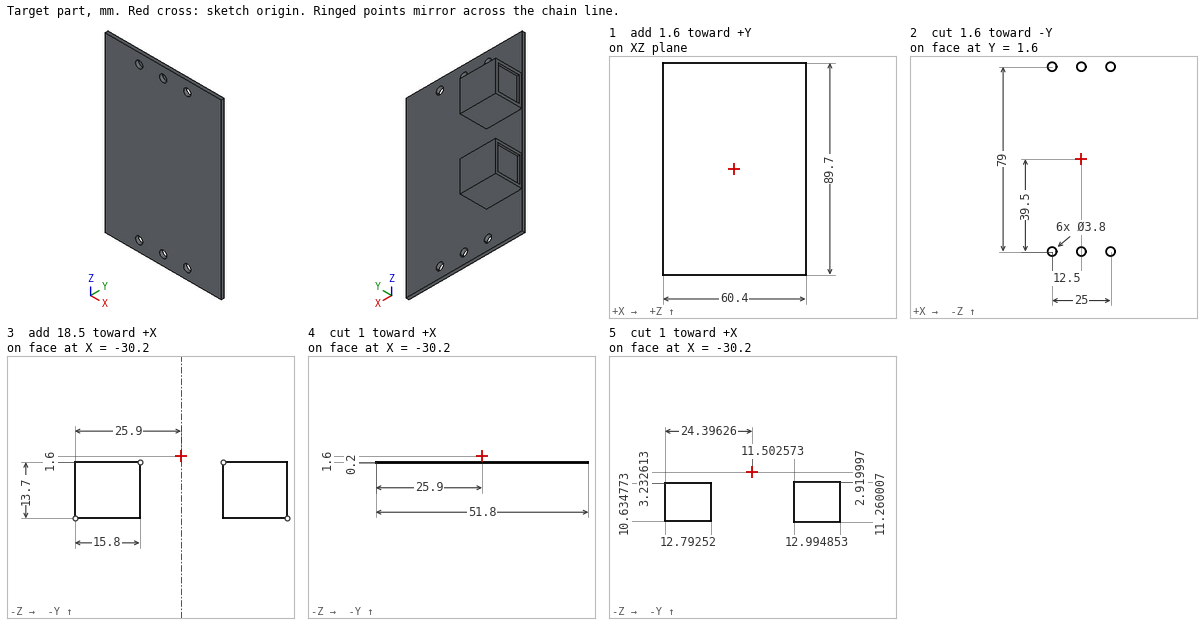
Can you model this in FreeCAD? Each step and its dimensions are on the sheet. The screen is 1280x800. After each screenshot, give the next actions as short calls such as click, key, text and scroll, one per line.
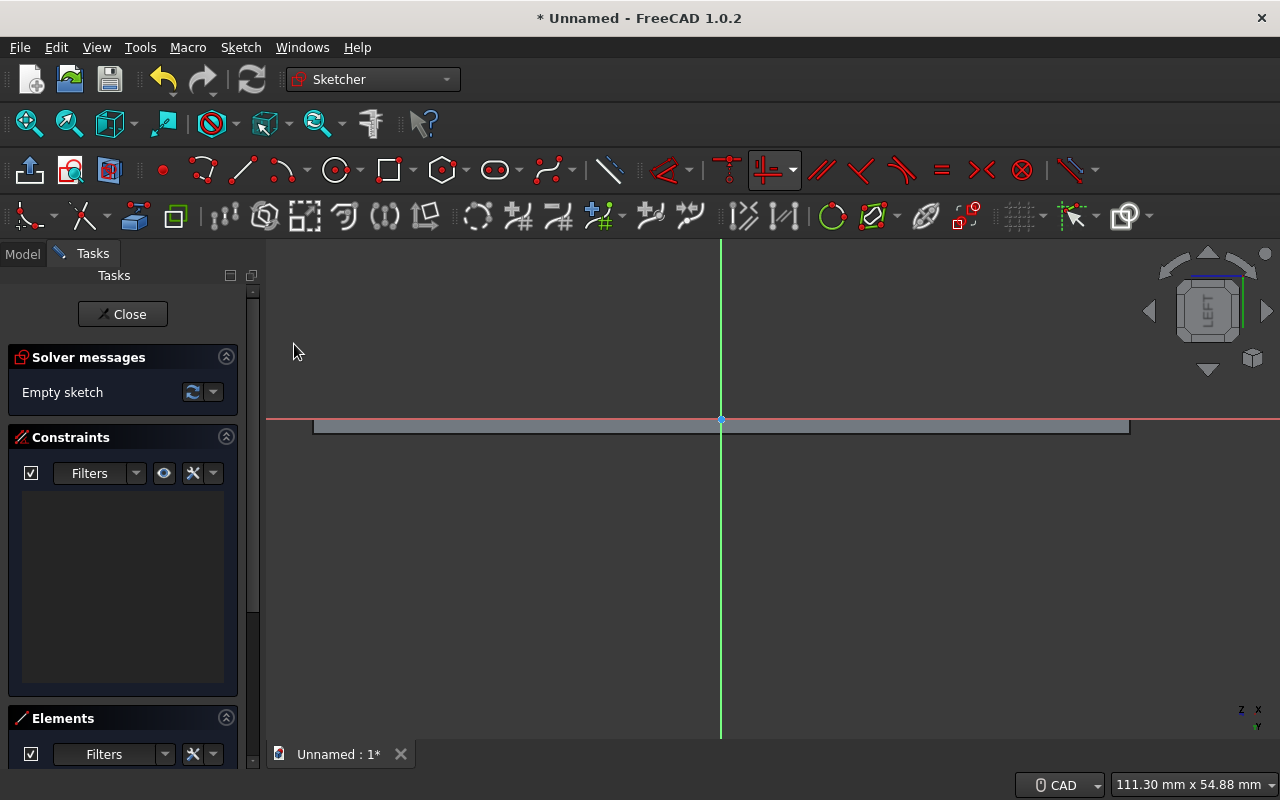
key(g)
key(r)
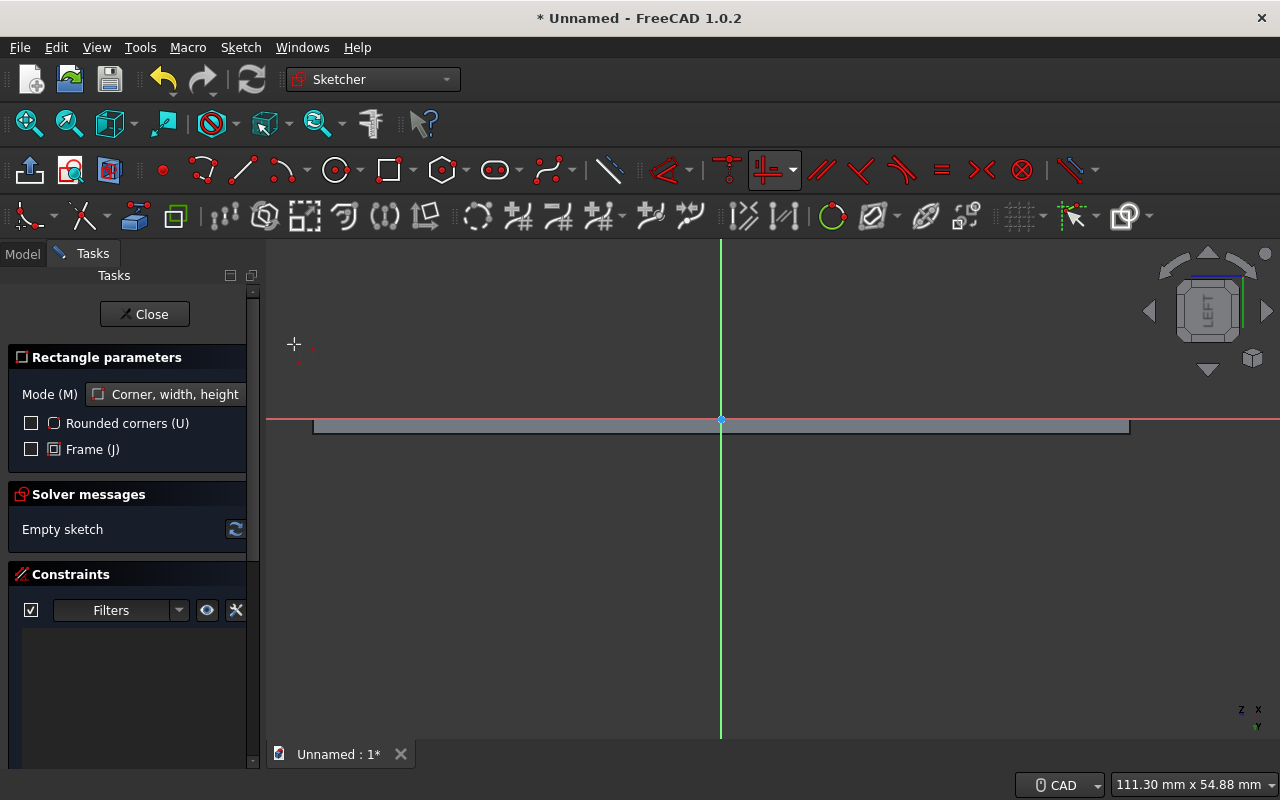
click(485, 434)
click(629, 559)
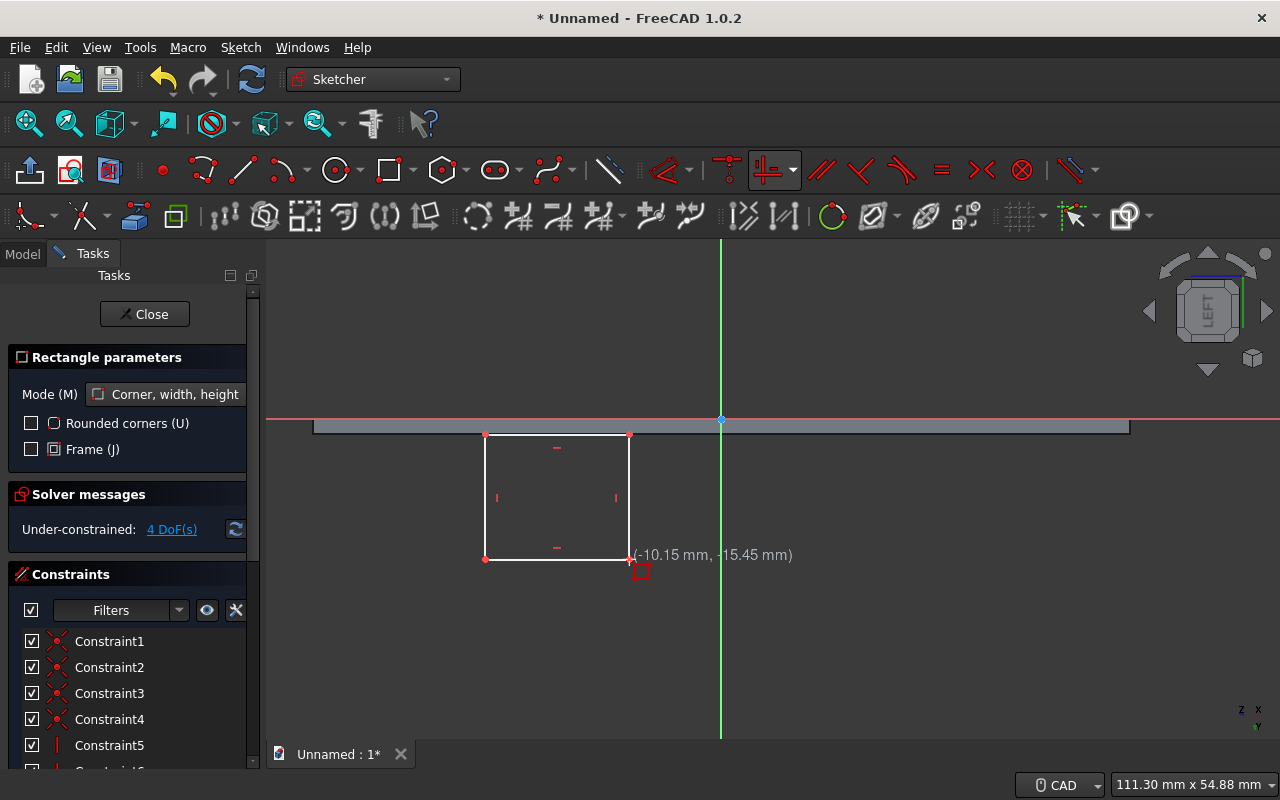
click(813, 434)
click(957, 559)
key(Escape)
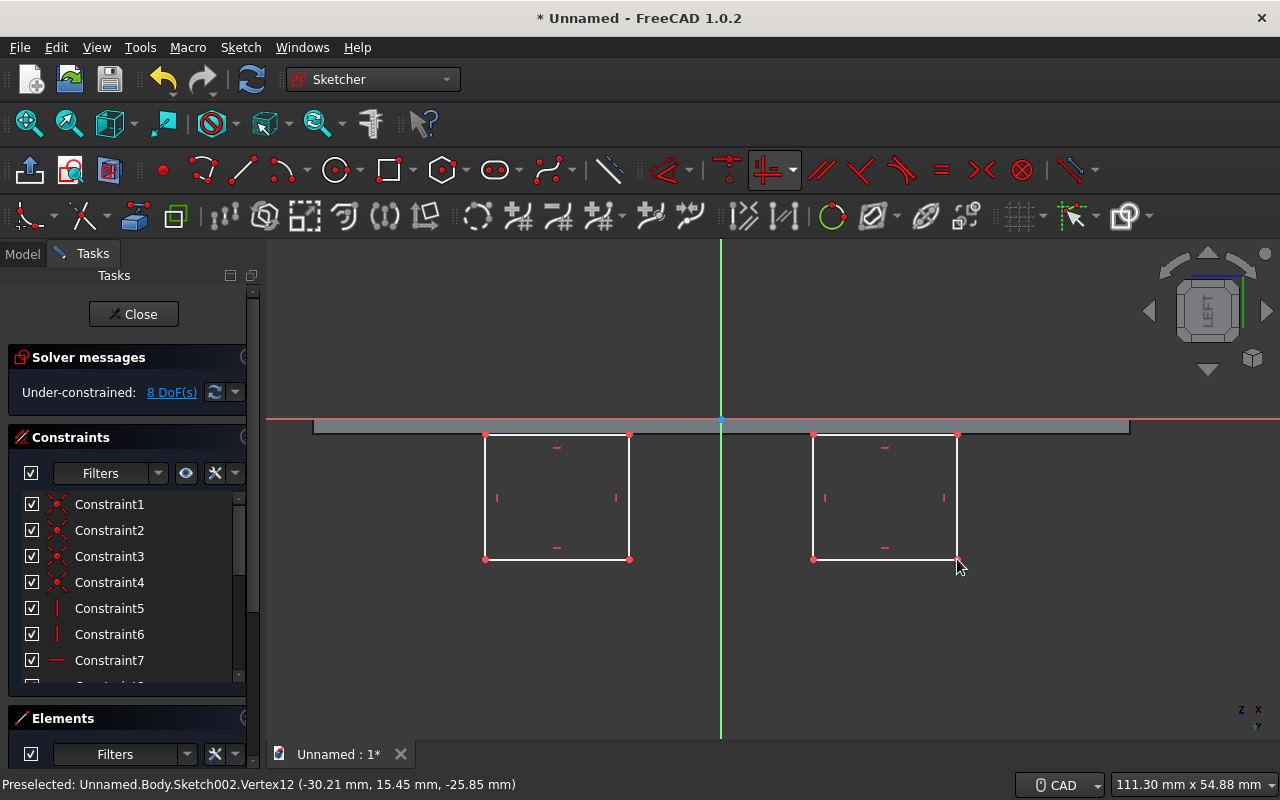
click(629, 435)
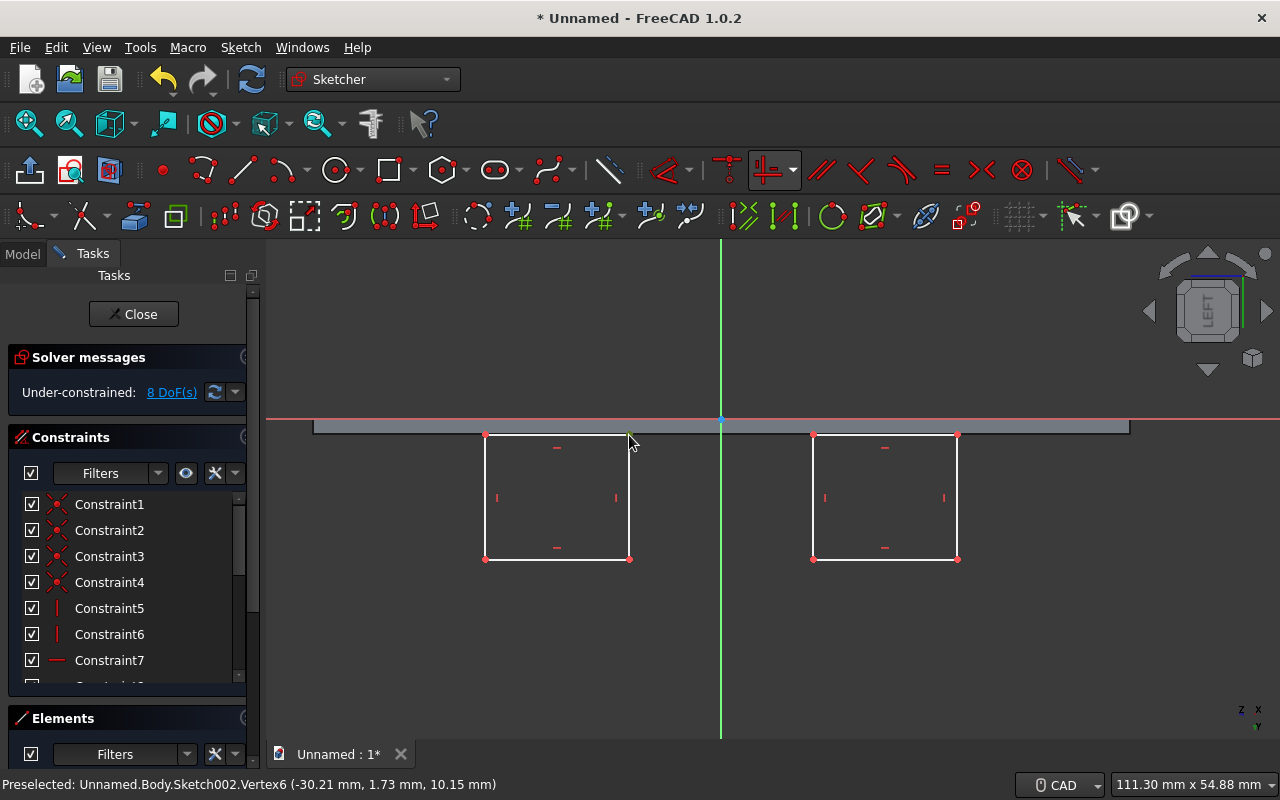
click(813, 435)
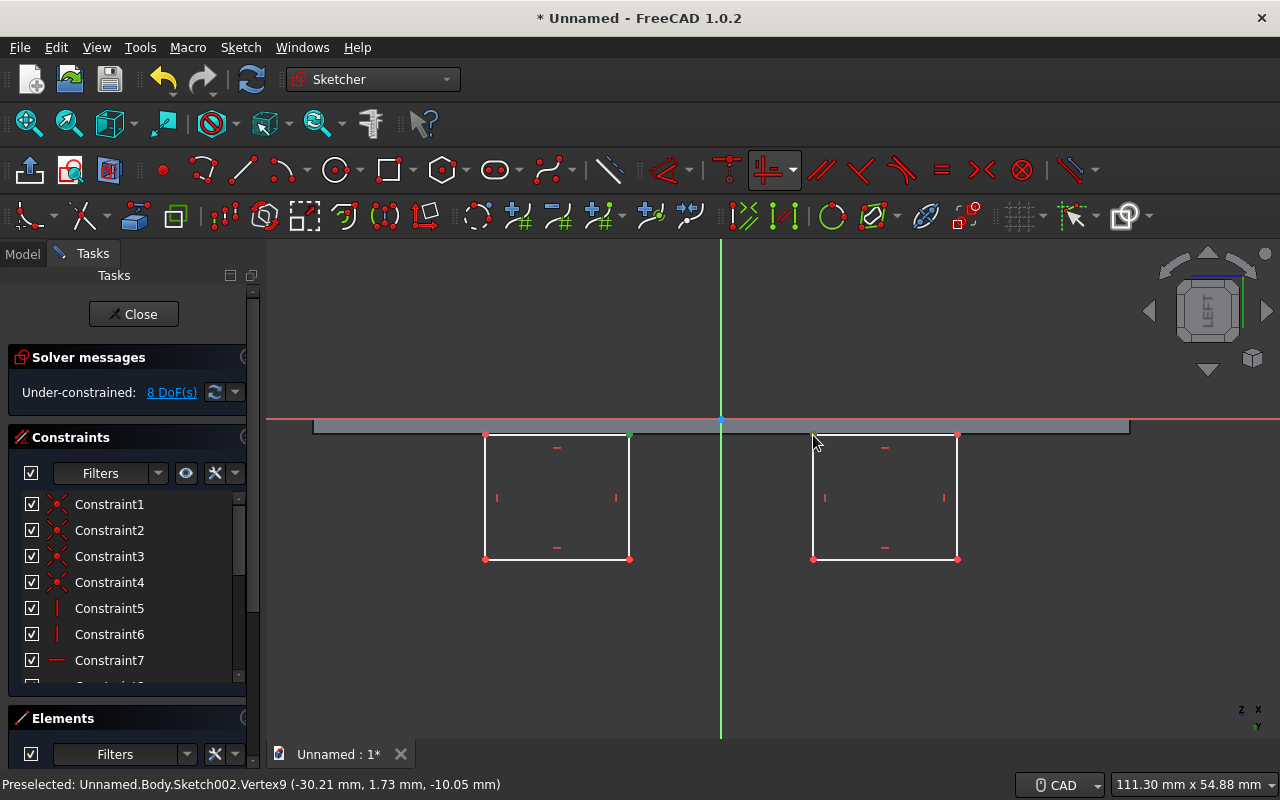
click(721, 679)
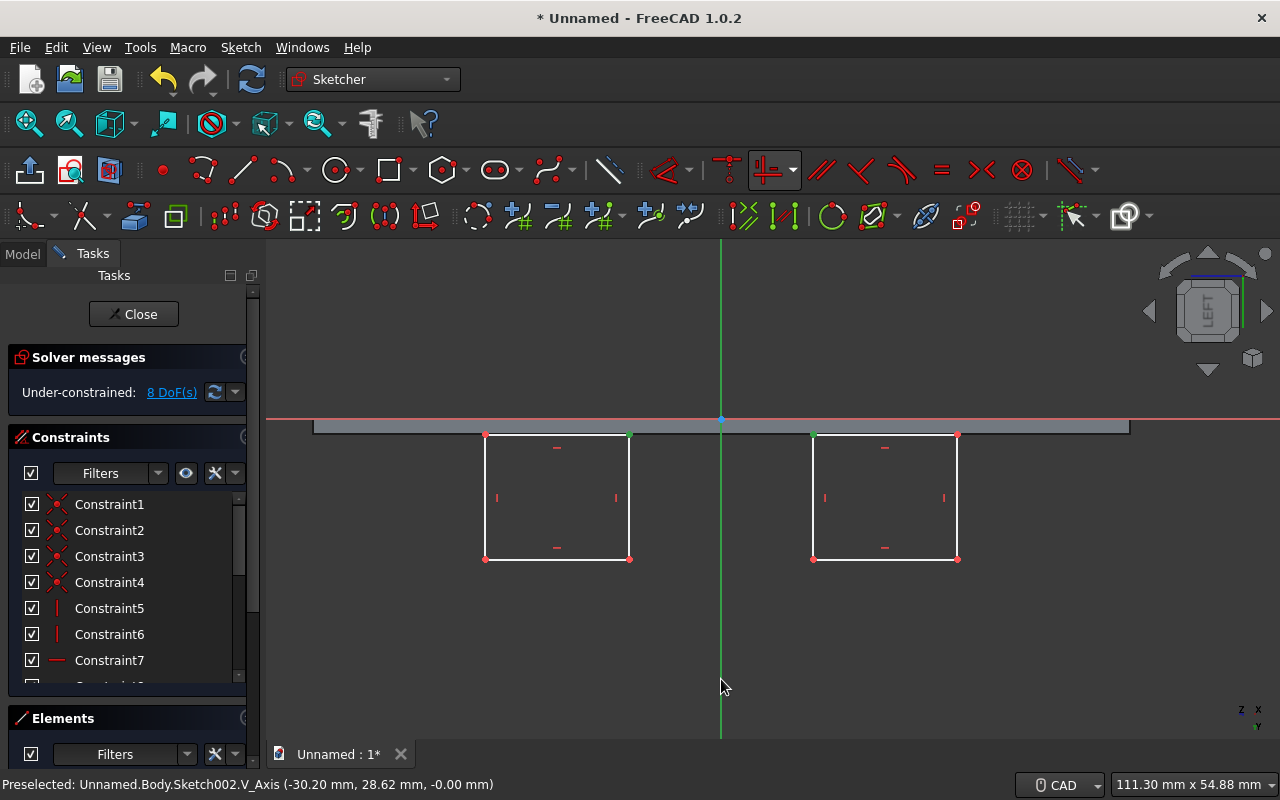
key(s)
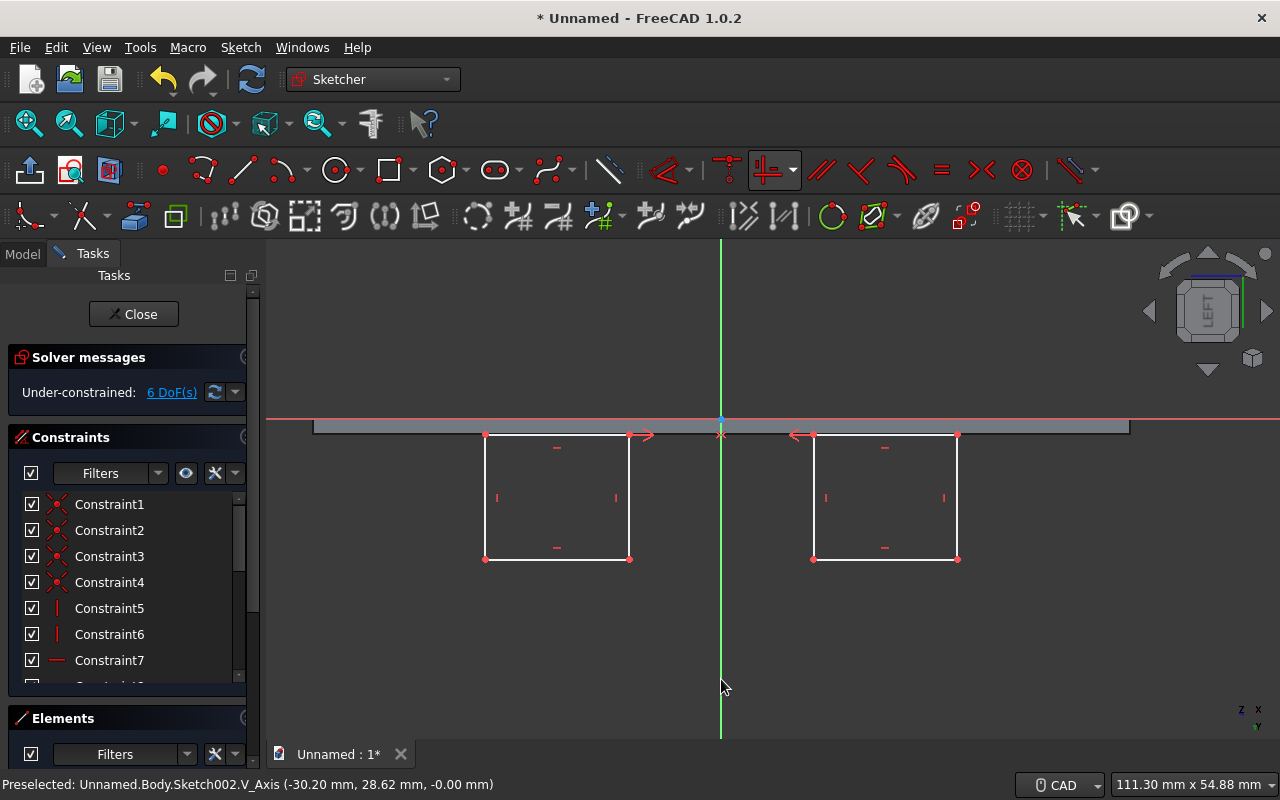
click(485, 560)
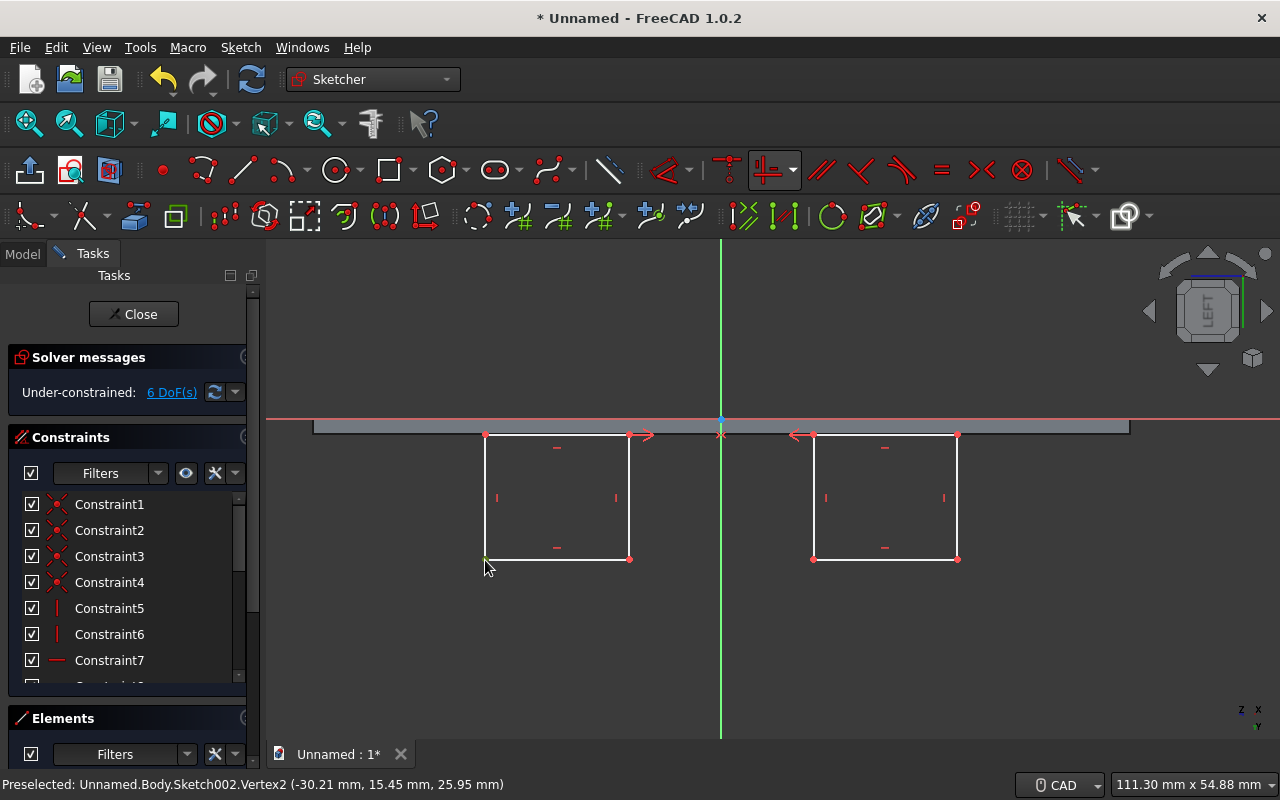
click(957, 560)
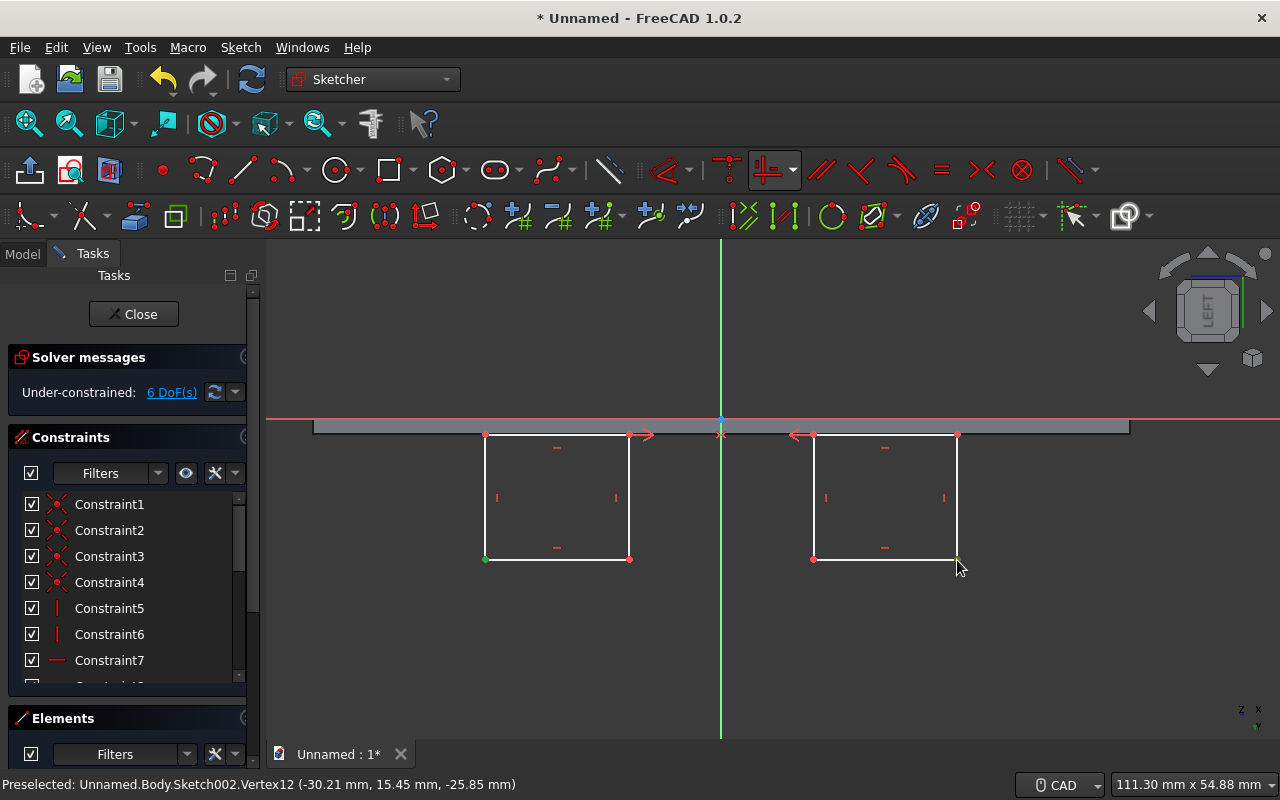
click(721, 679)